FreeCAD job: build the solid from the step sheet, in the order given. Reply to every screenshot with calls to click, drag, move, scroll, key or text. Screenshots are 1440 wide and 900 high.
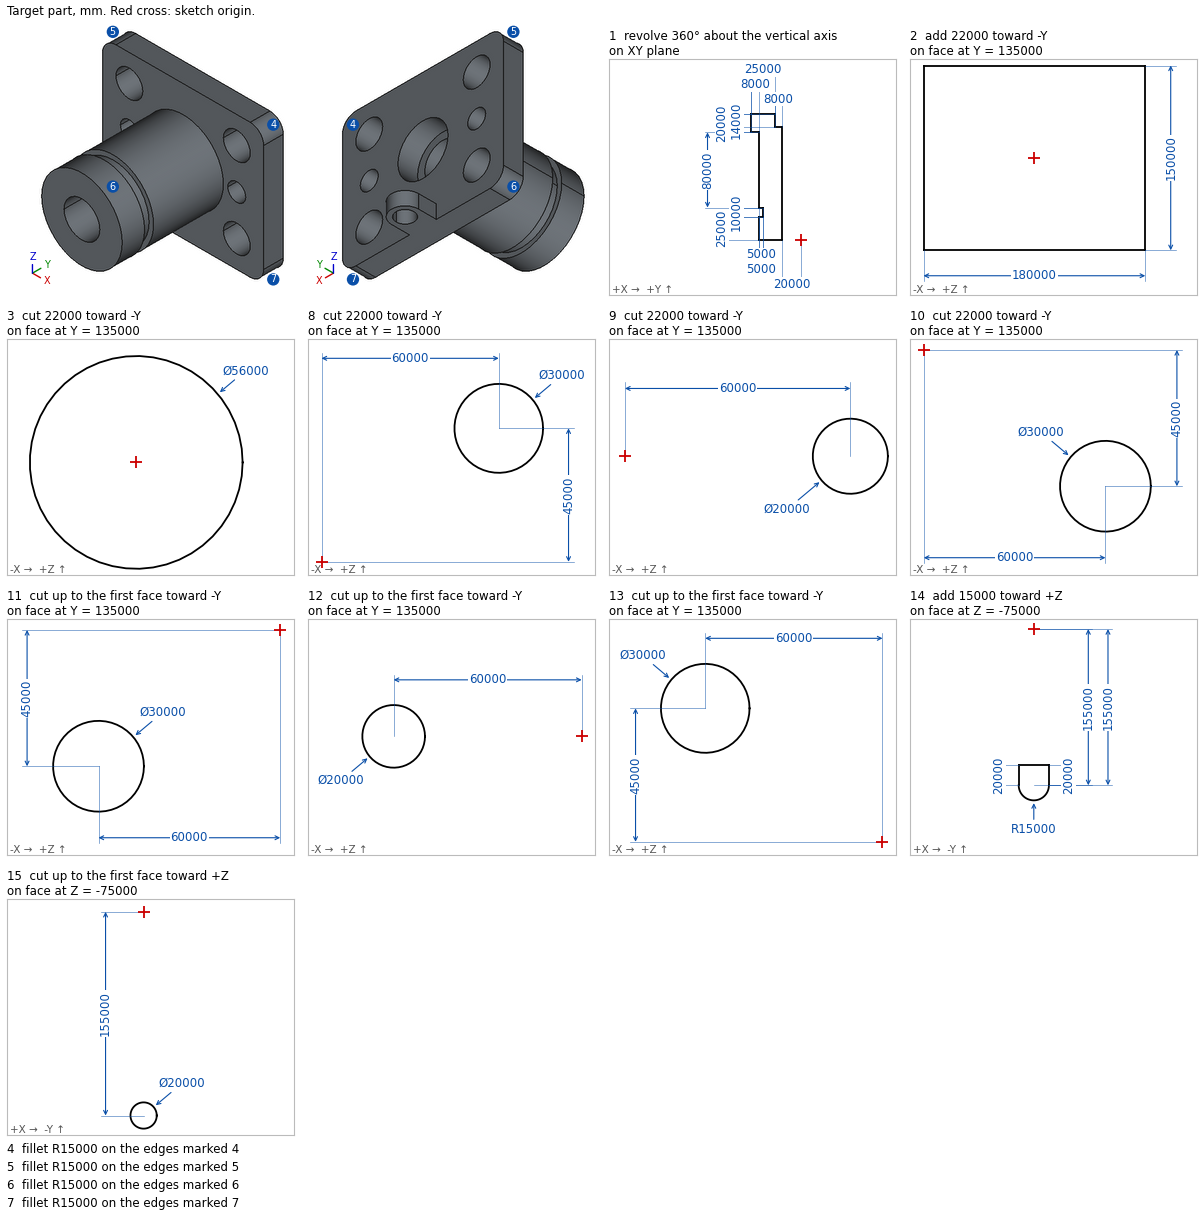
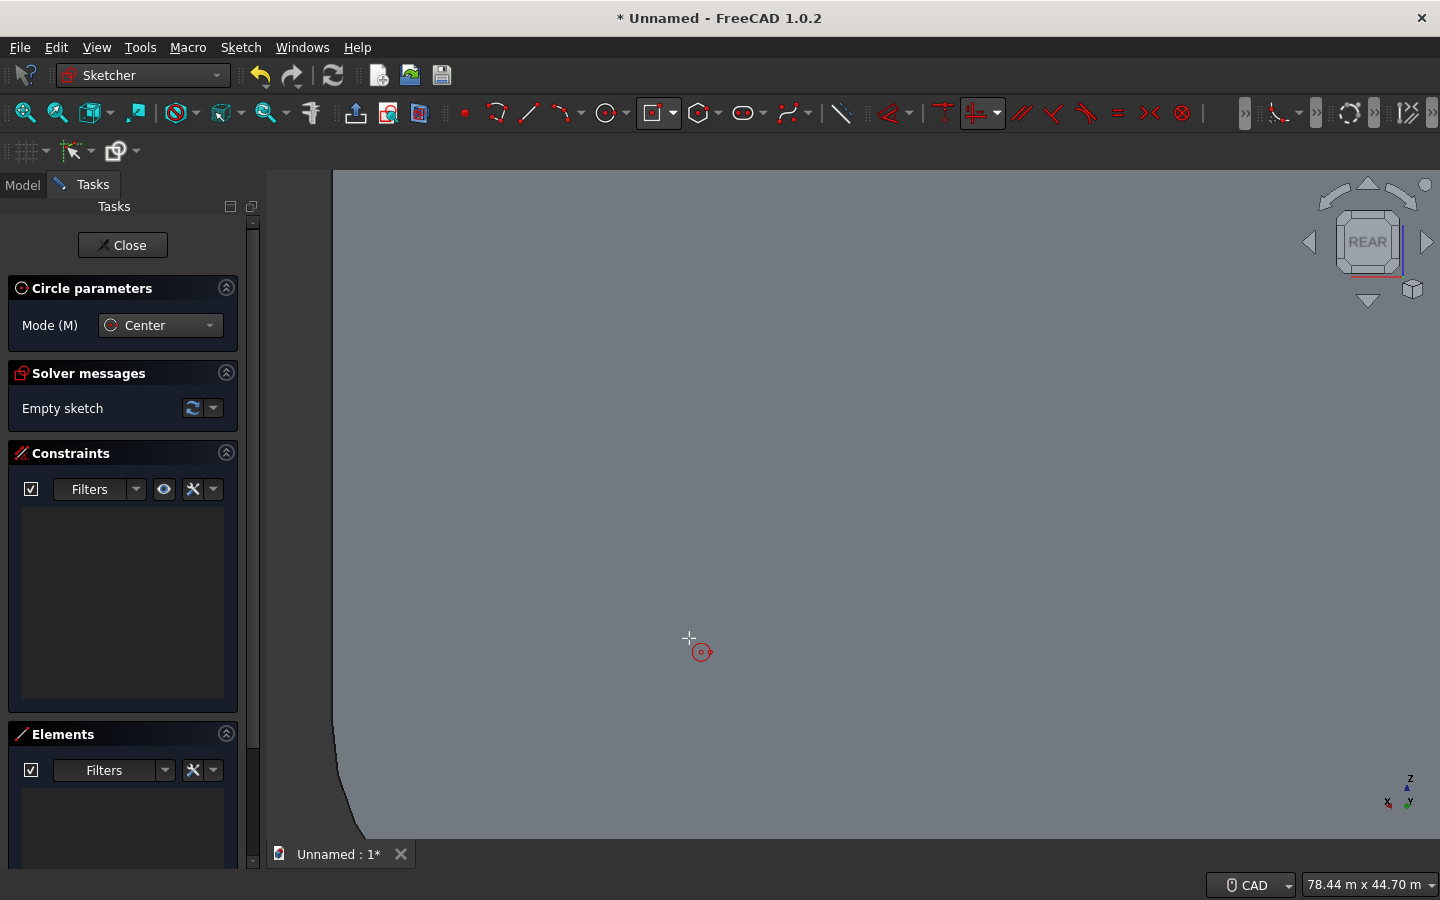
click(781, 500)
click(940, 342)
key(Escape)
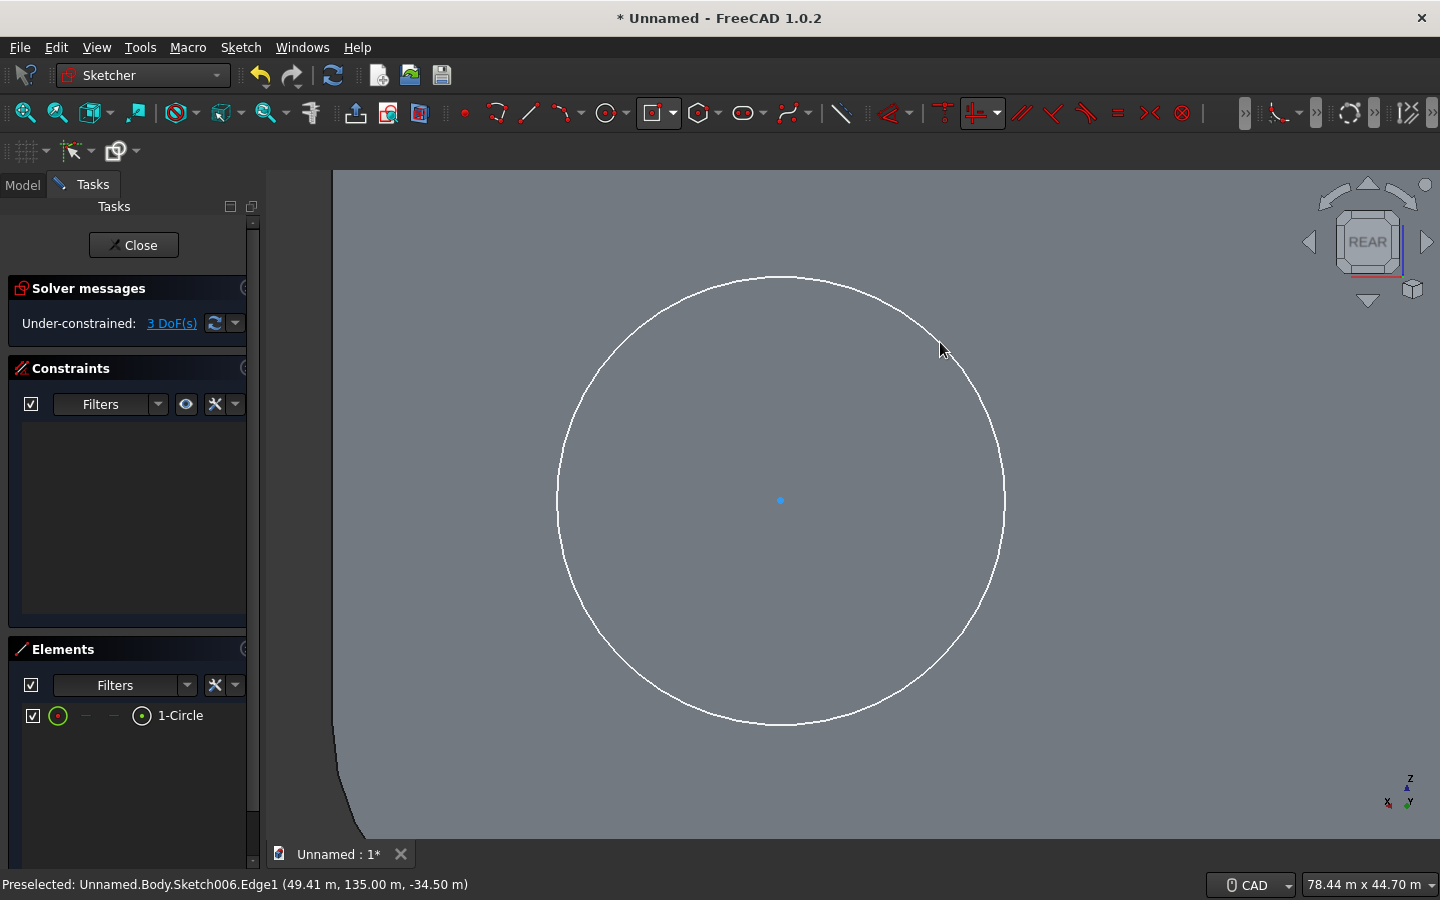
click(888, 114)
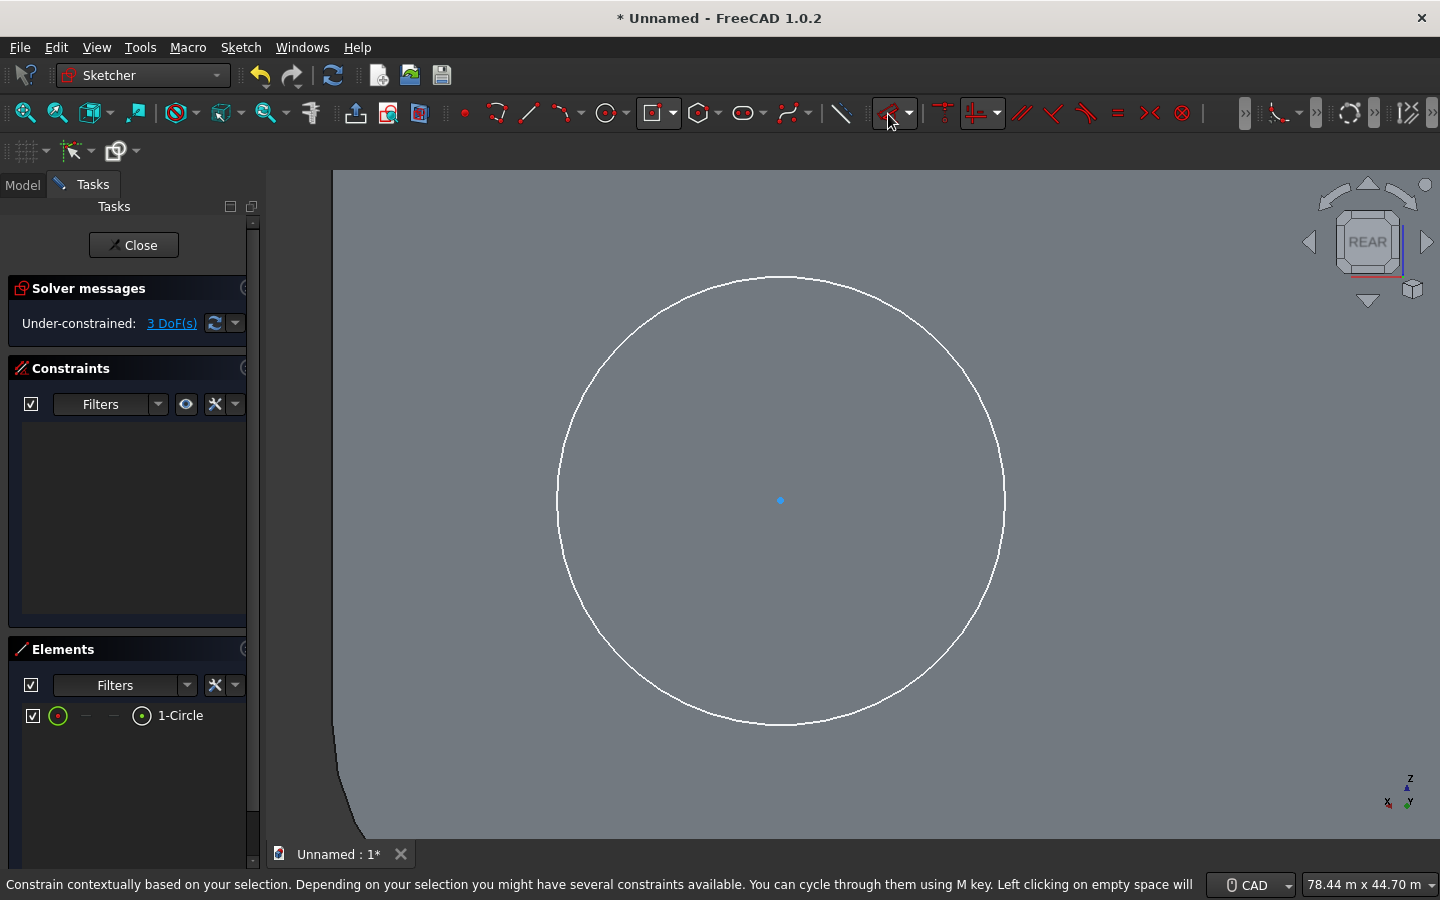
click(939, 342)
click(962, 319)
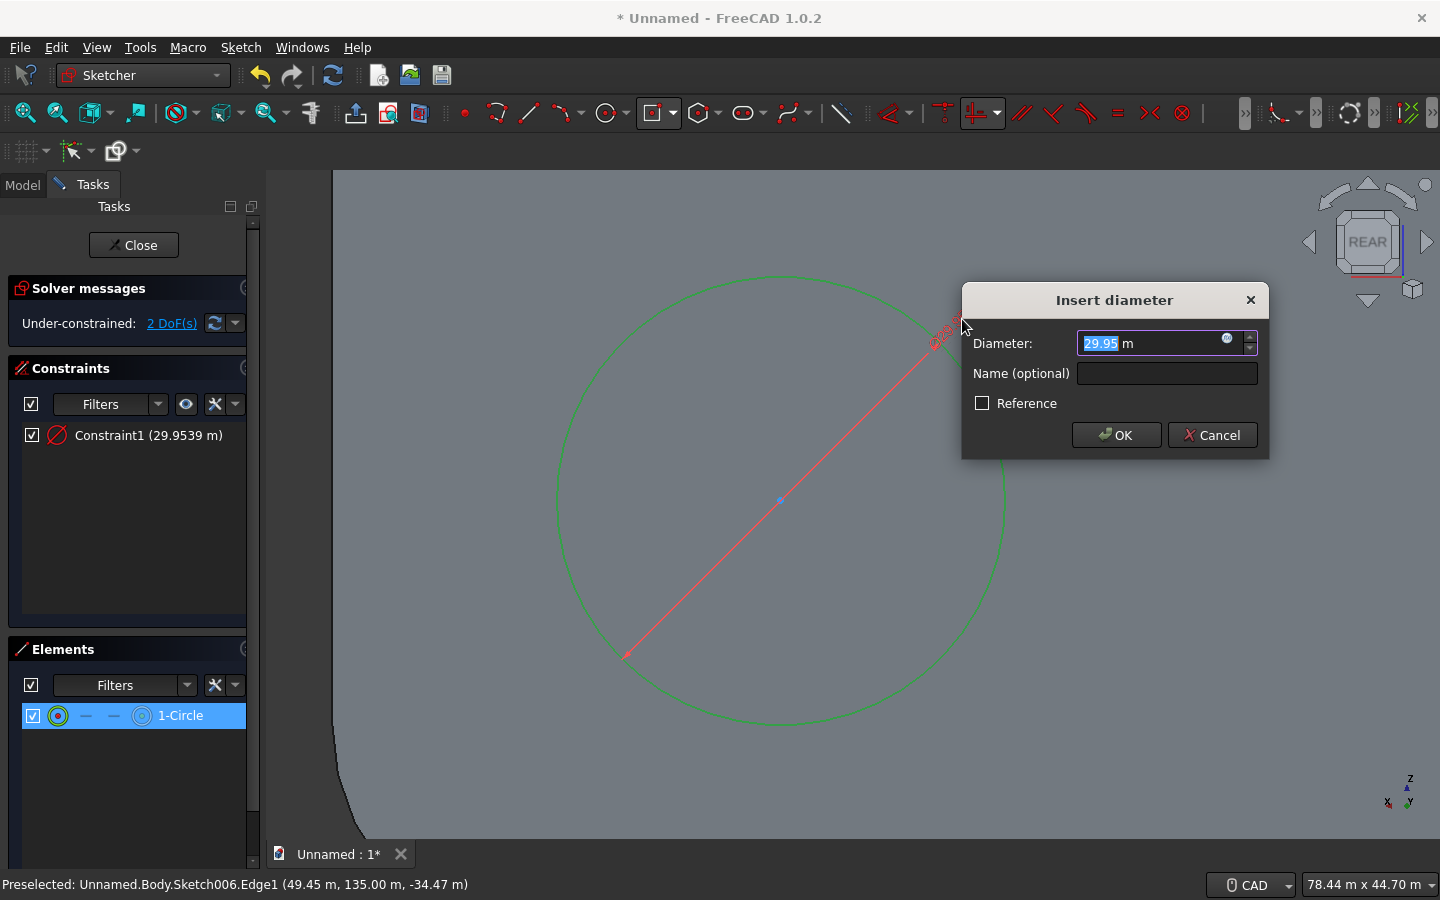
key(ctrl+a)
text(30000 mm)
key(Return)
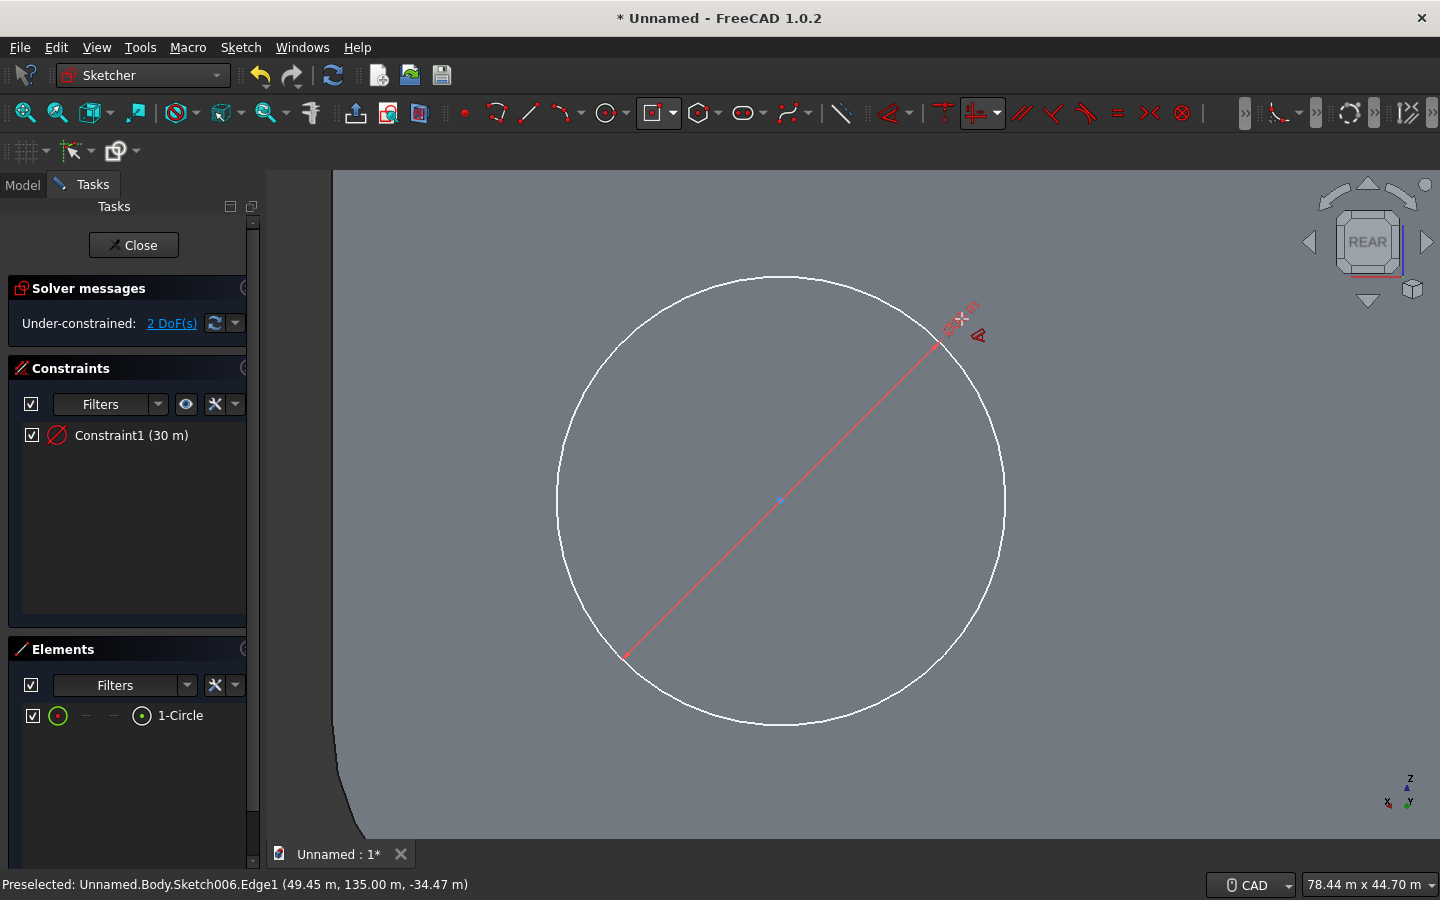
click(781, 501)
click(1028, 535)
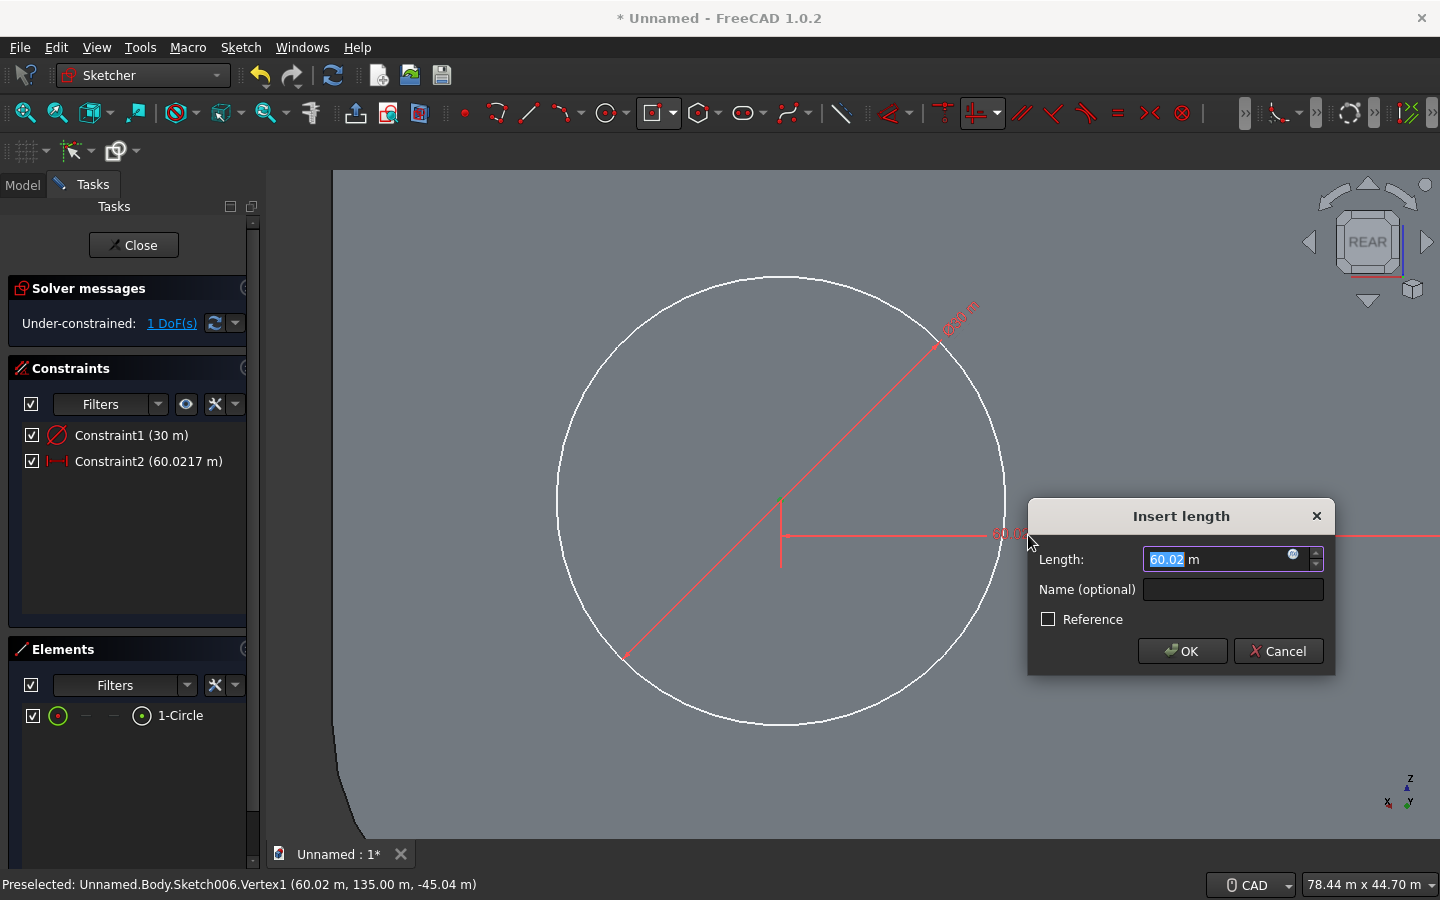
key(ctrl+a)
text(60000 mm)
key(Return)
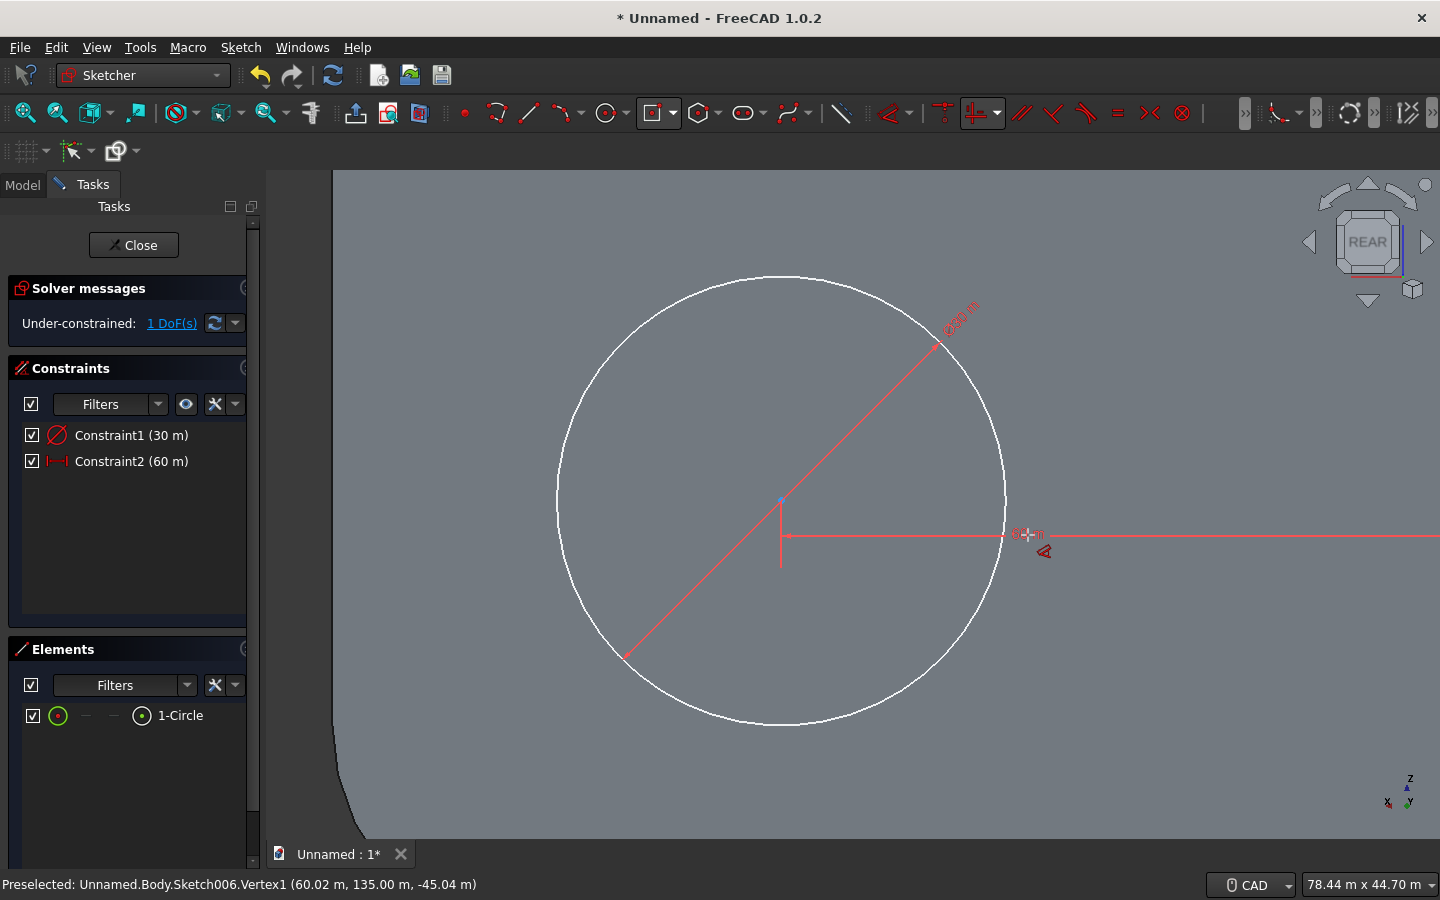
click(781, 501)
click(747, 349)